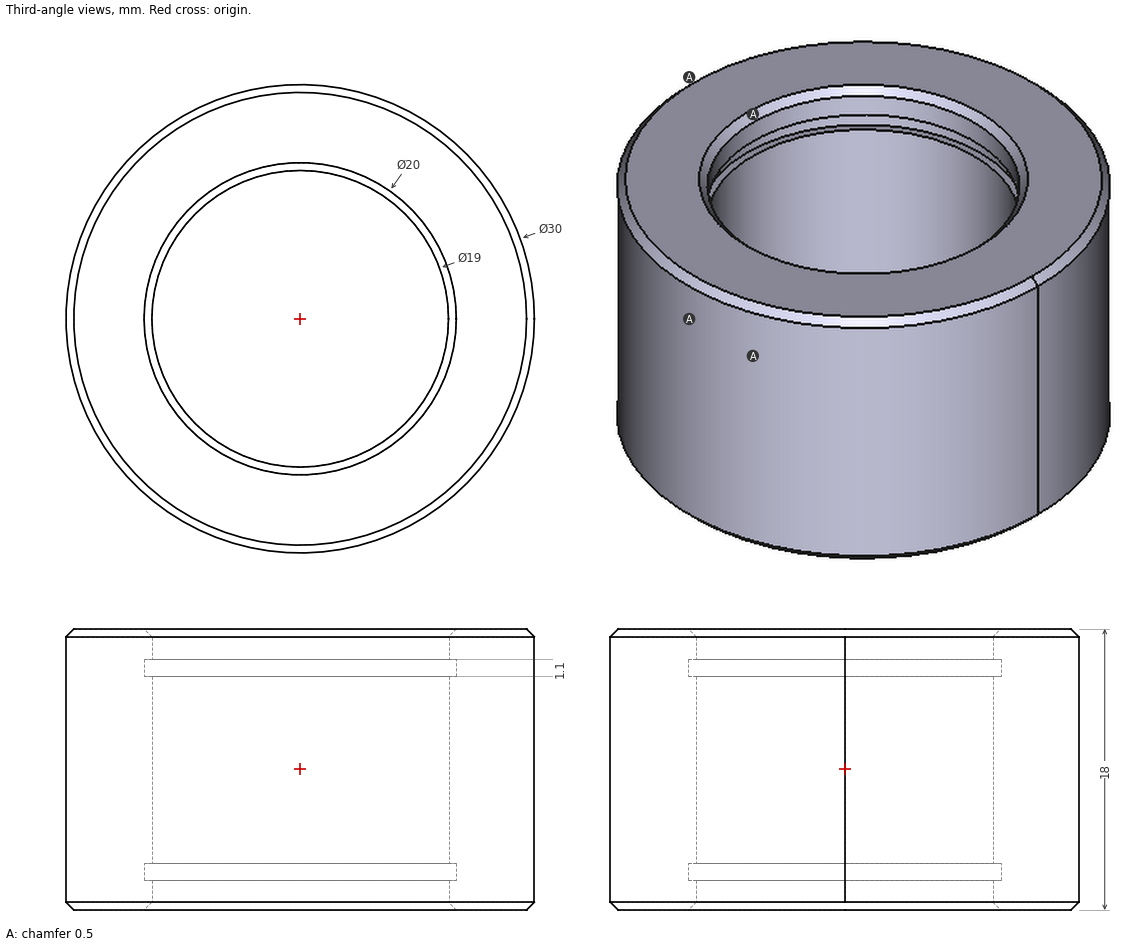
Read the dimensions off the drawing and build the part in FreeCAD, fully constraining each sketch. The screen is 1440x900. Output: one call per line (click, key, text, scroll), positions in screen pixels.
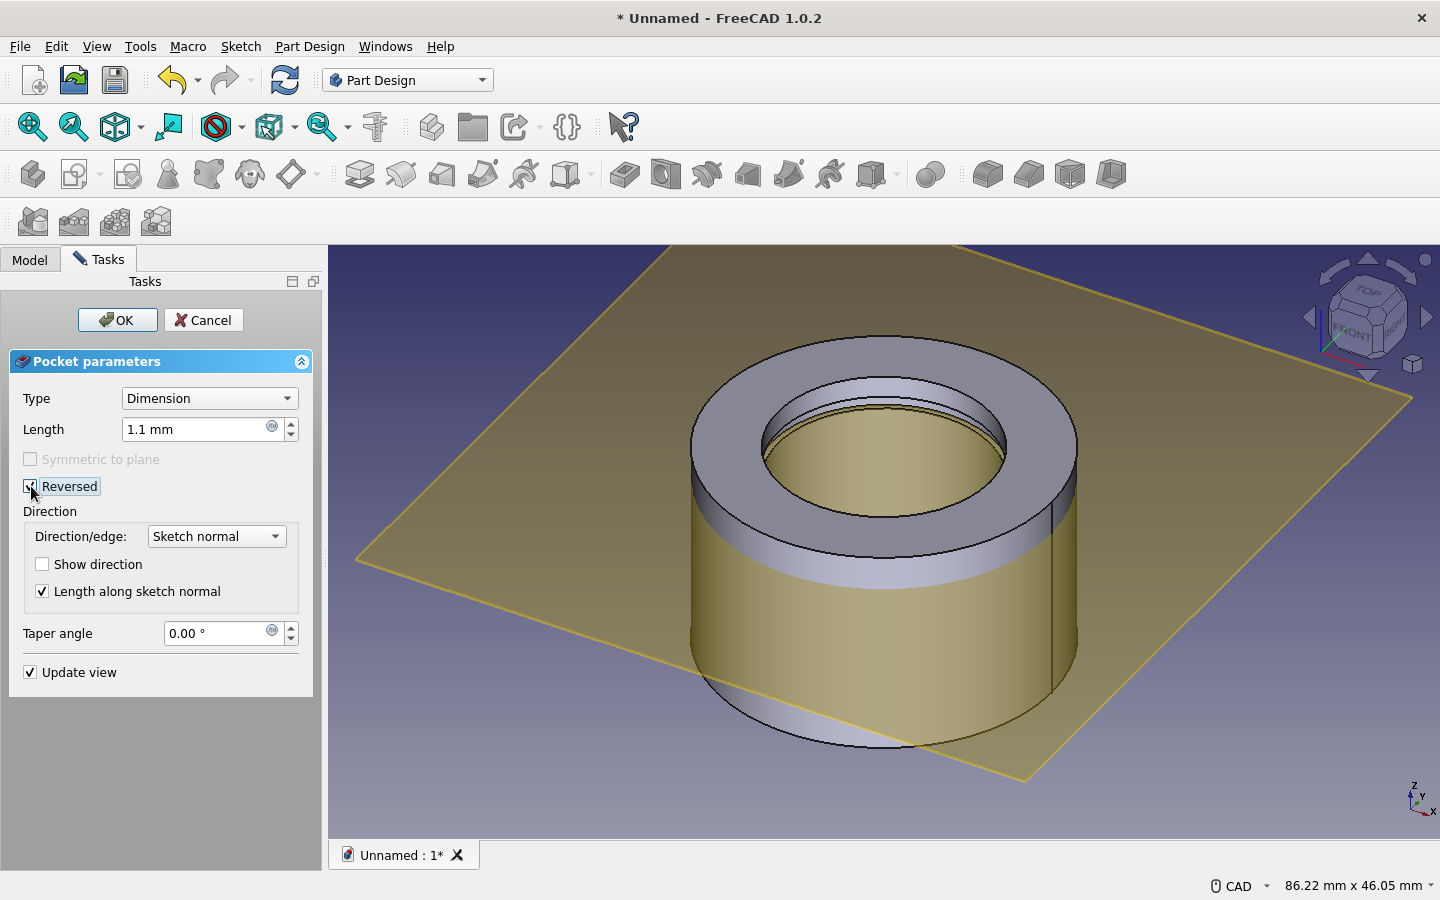
click(118, 320)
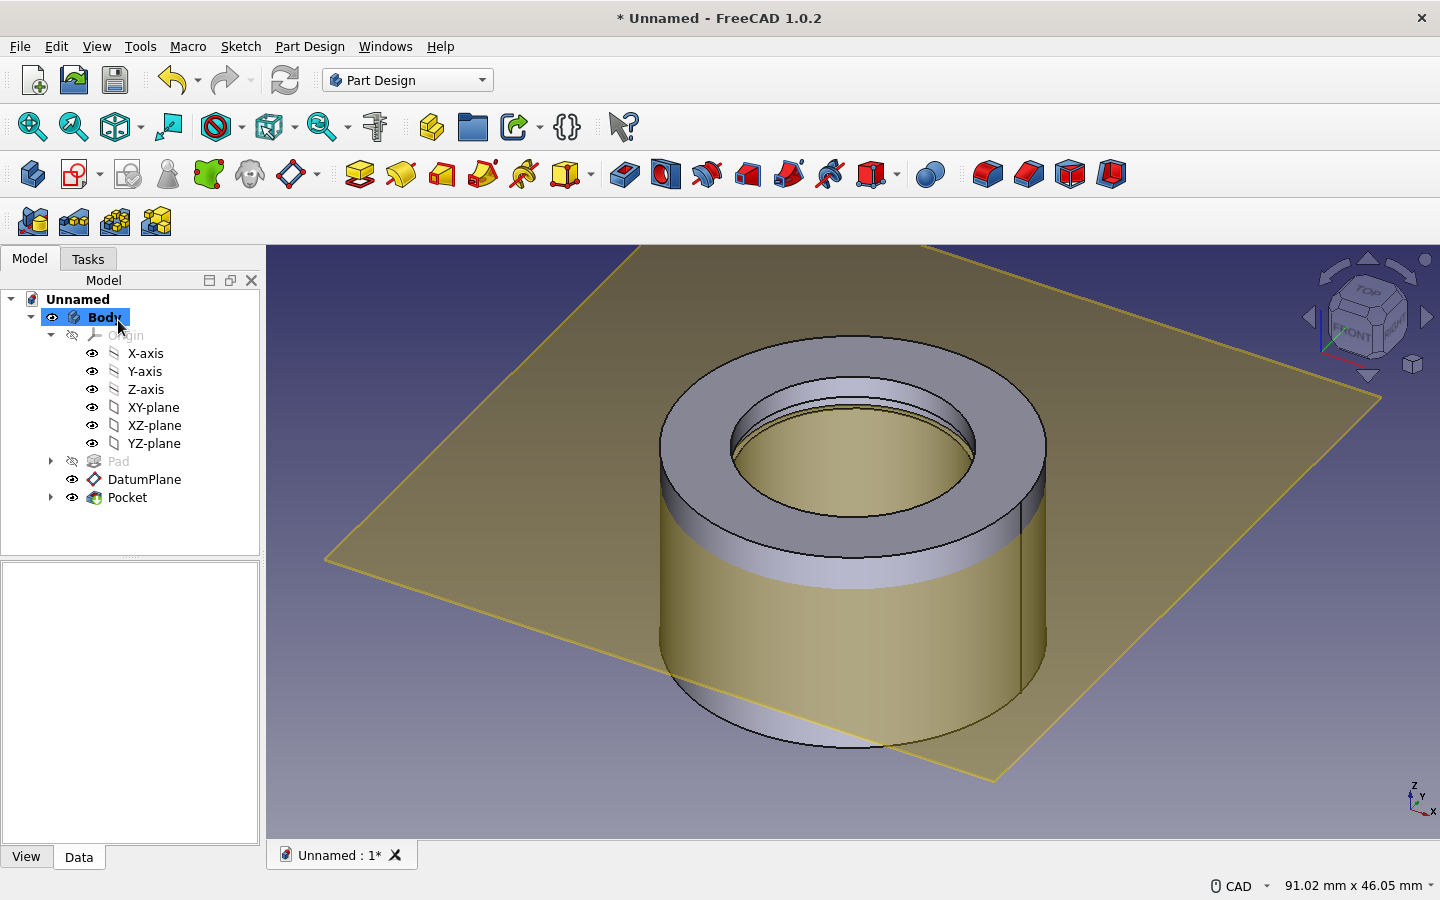
click(117, 479)
key(space)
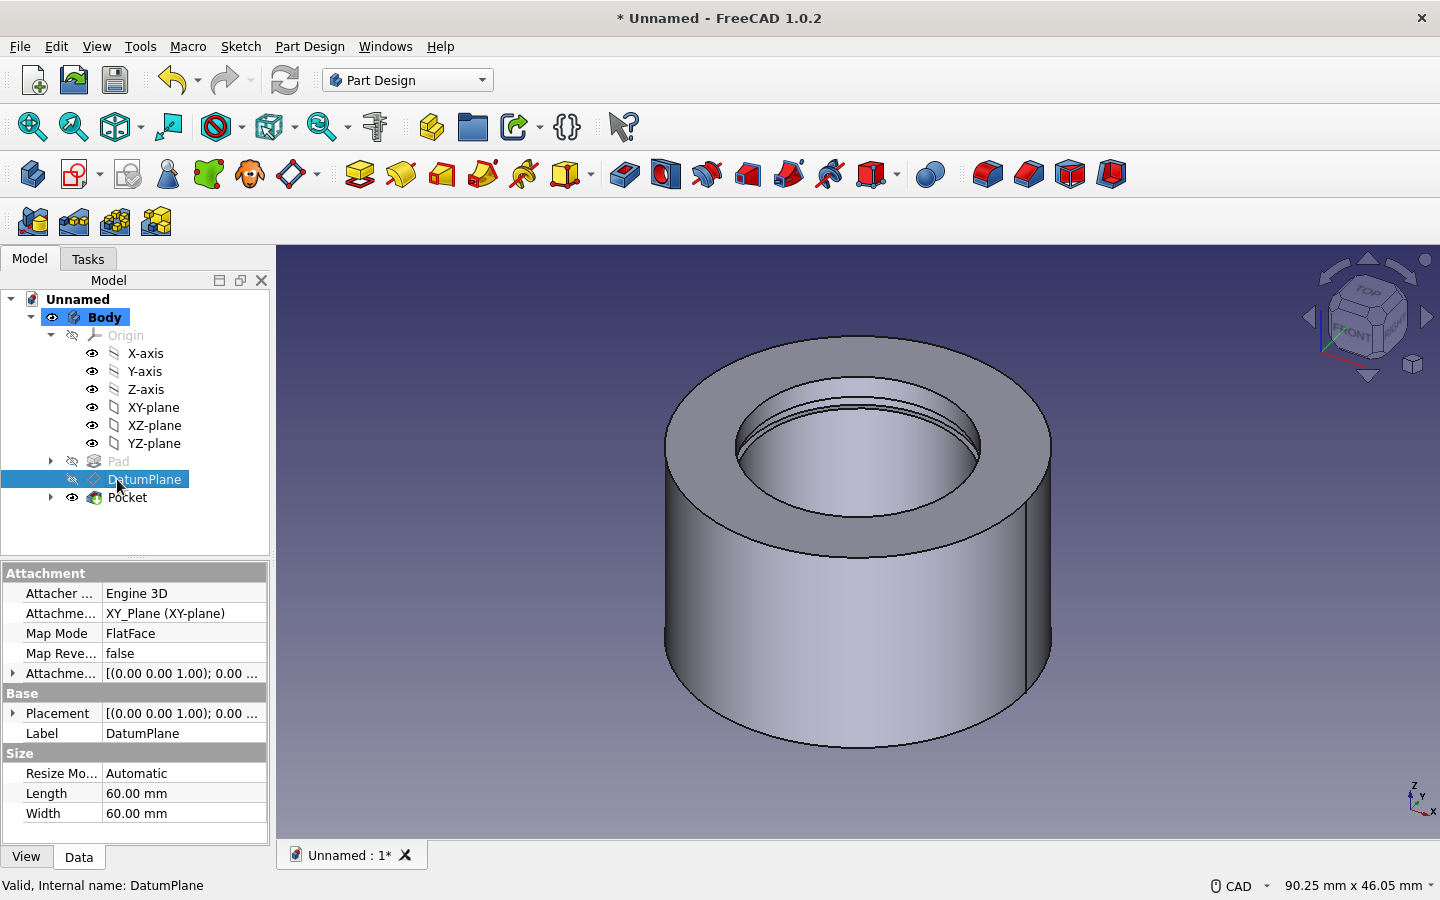
click(117, 497)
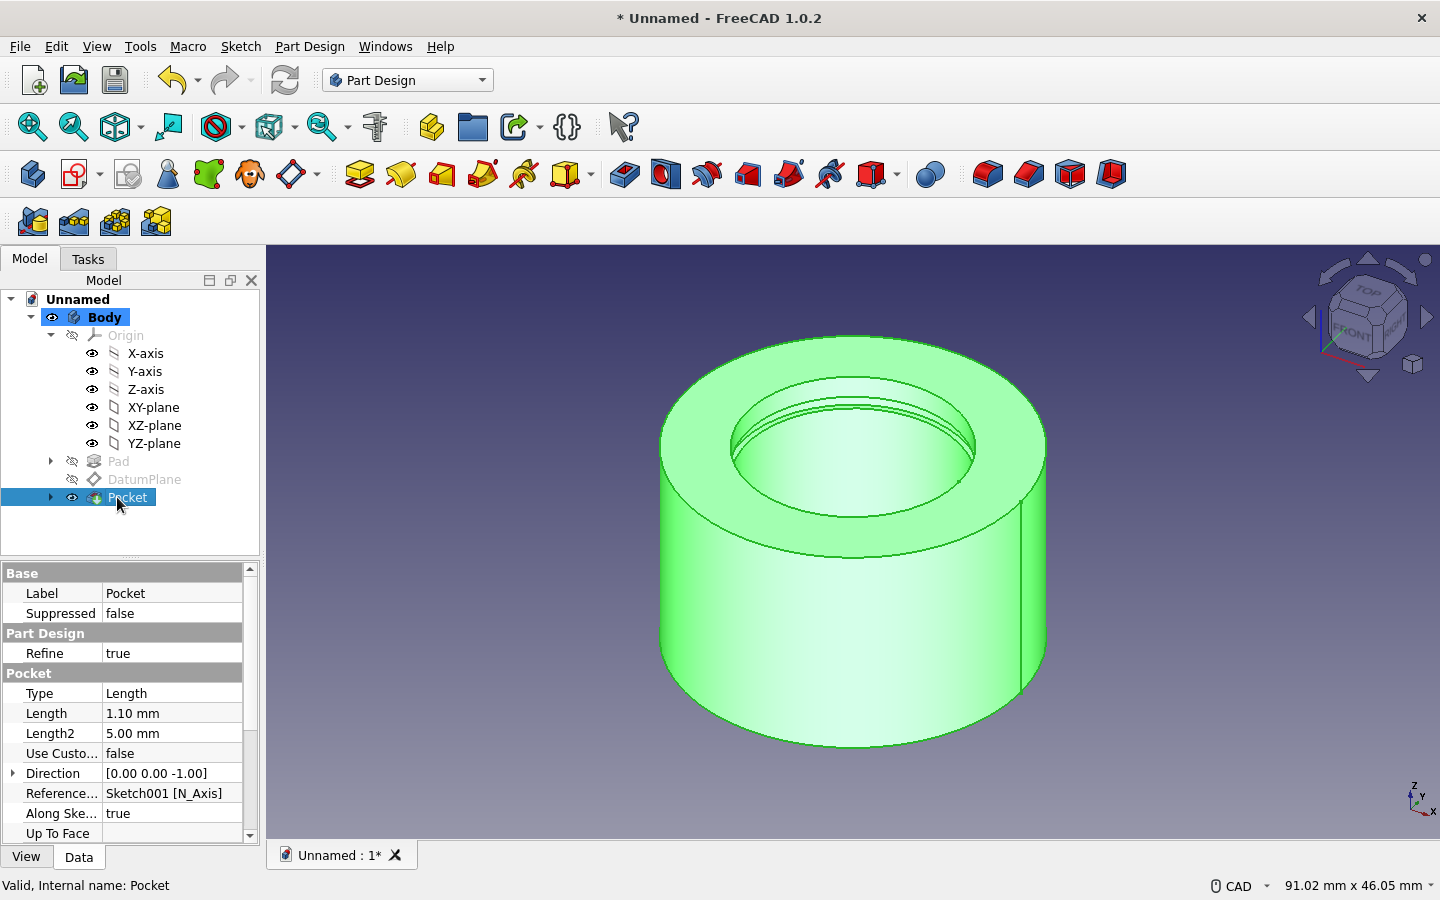
click(33, 222)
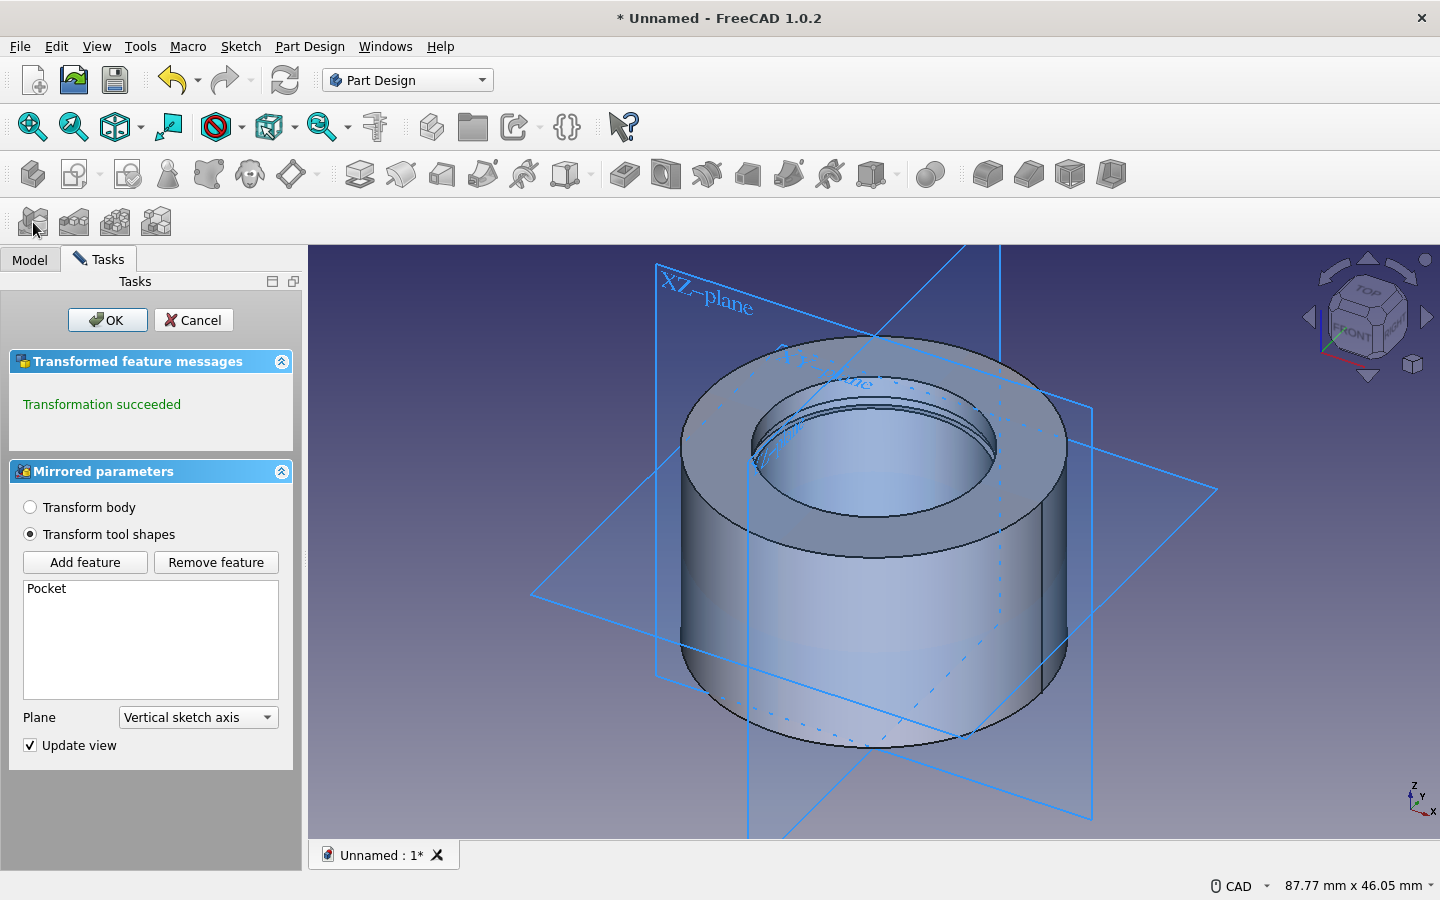
click(199, 718)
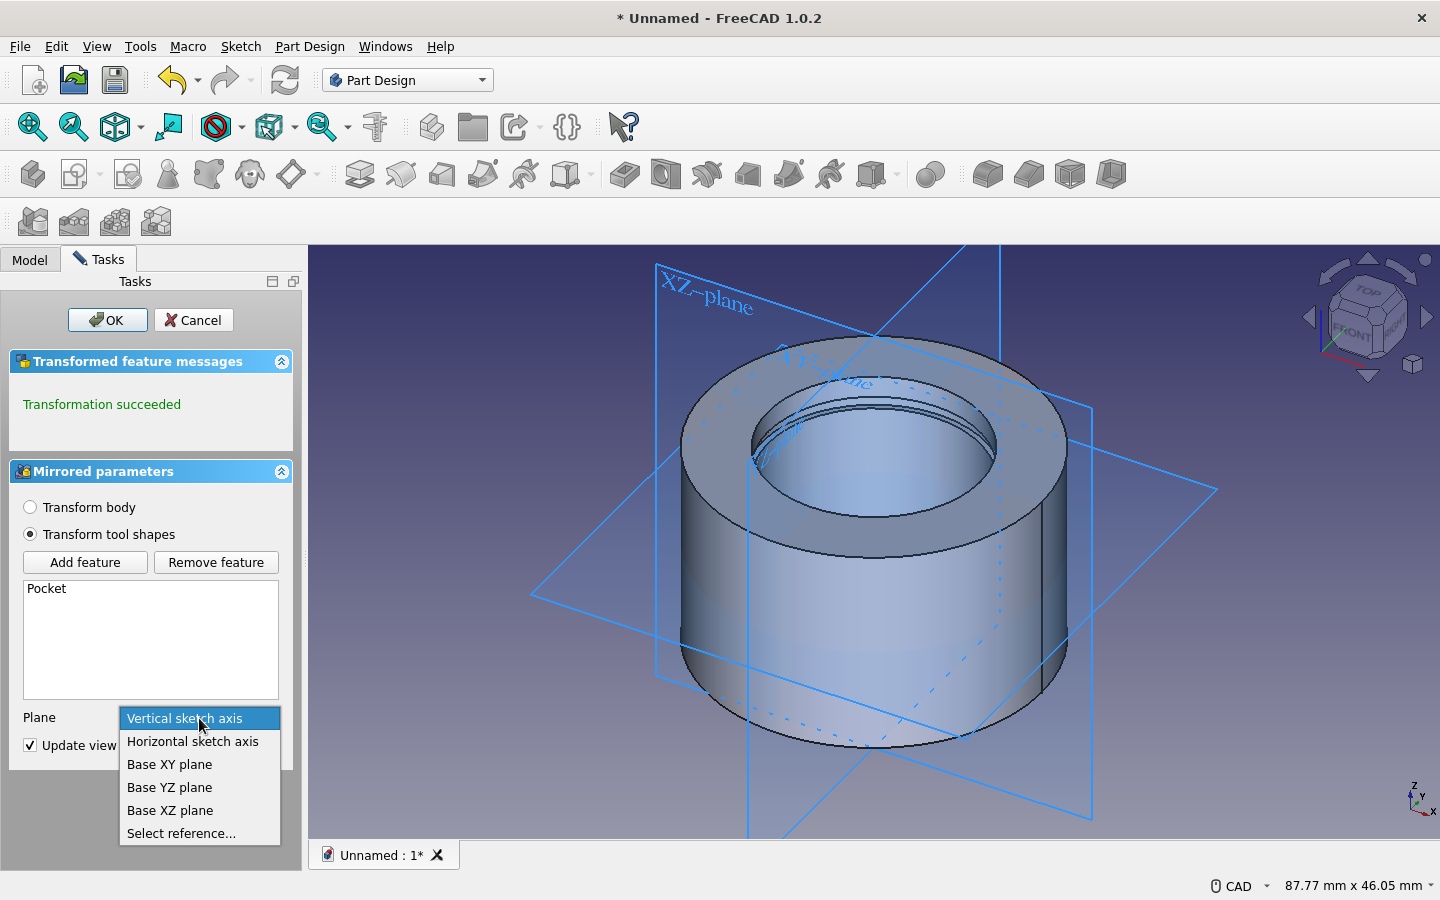
click(198, 764)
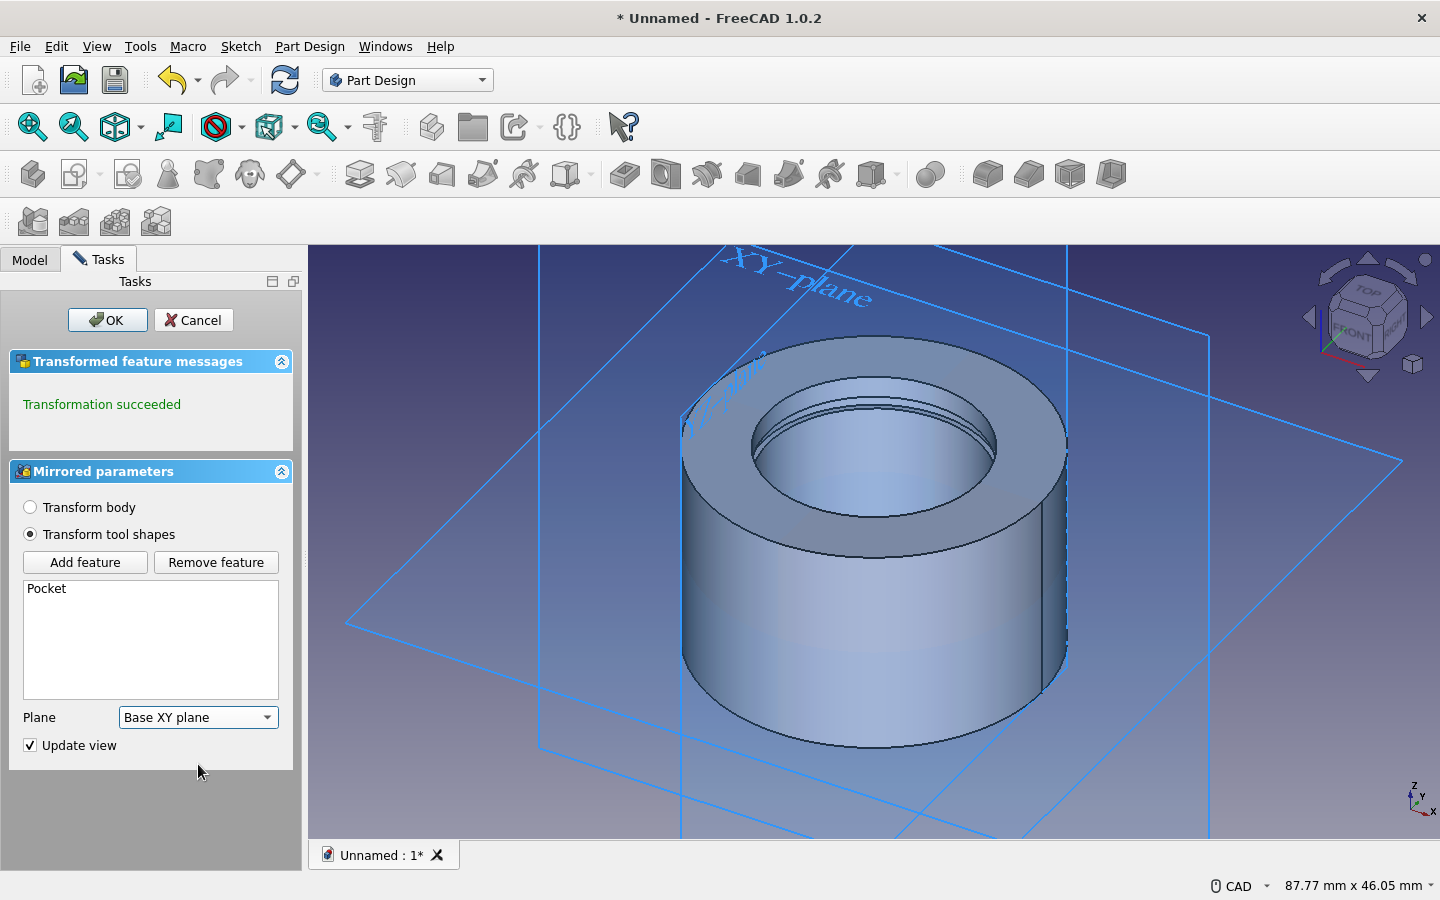
click(108, 320)